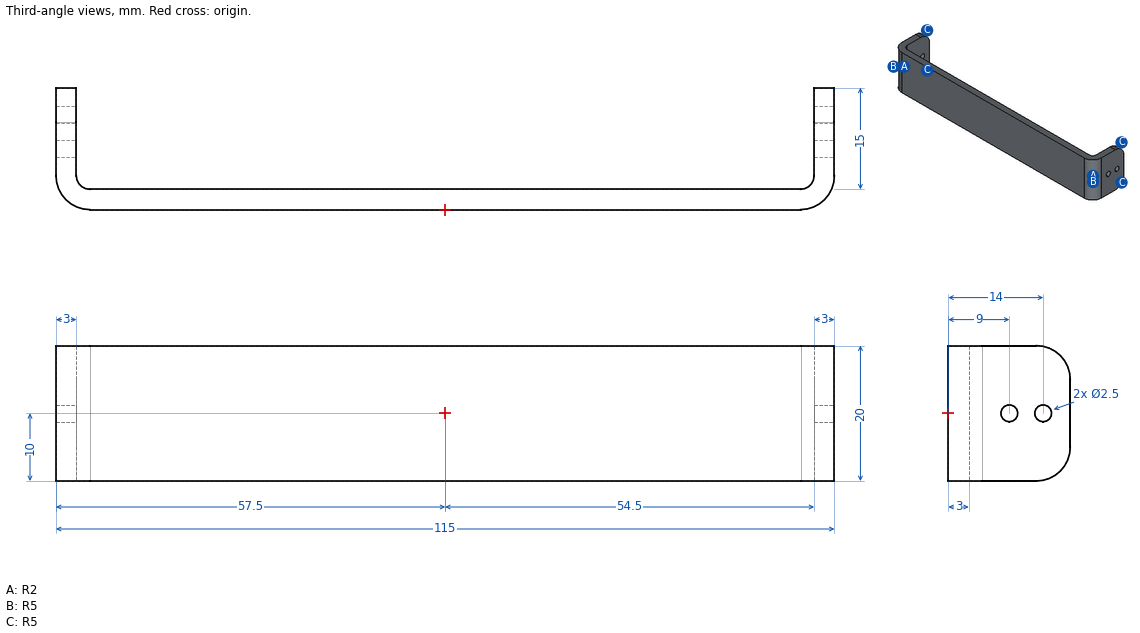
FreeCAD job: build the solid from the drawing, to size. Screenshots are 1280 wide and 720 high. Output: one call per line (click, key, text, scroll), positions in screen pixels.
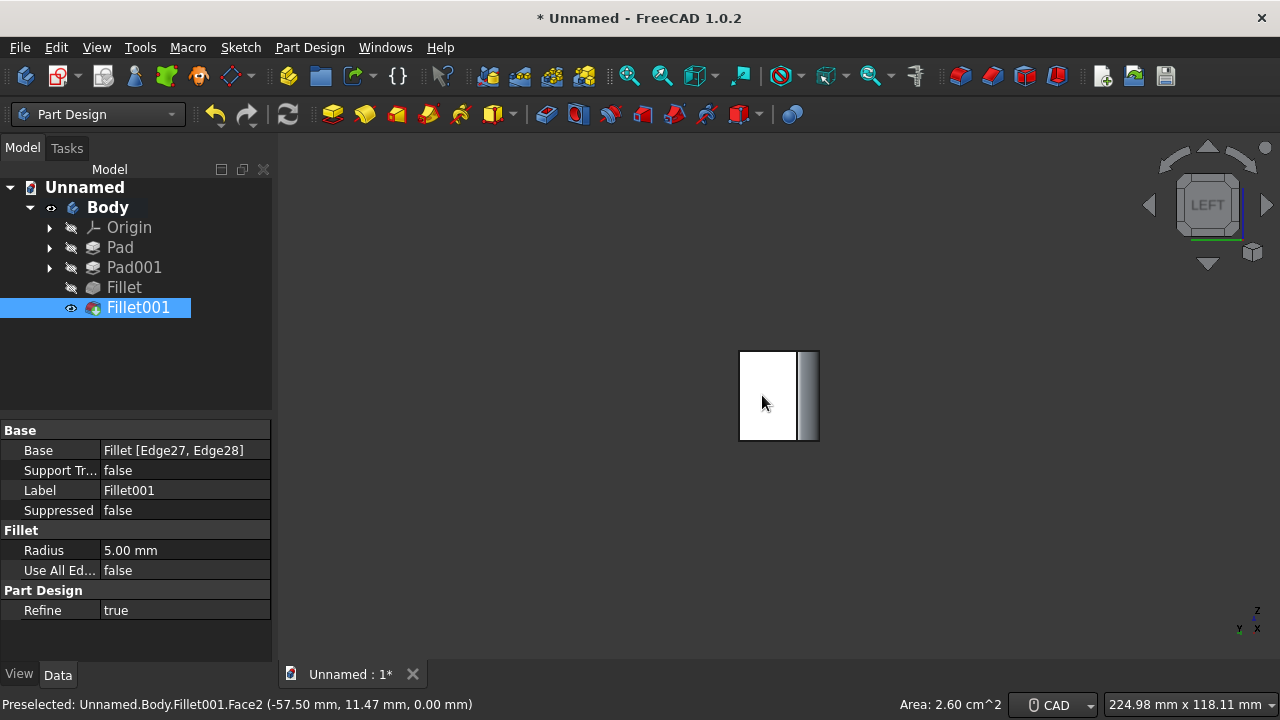
click(58, 76)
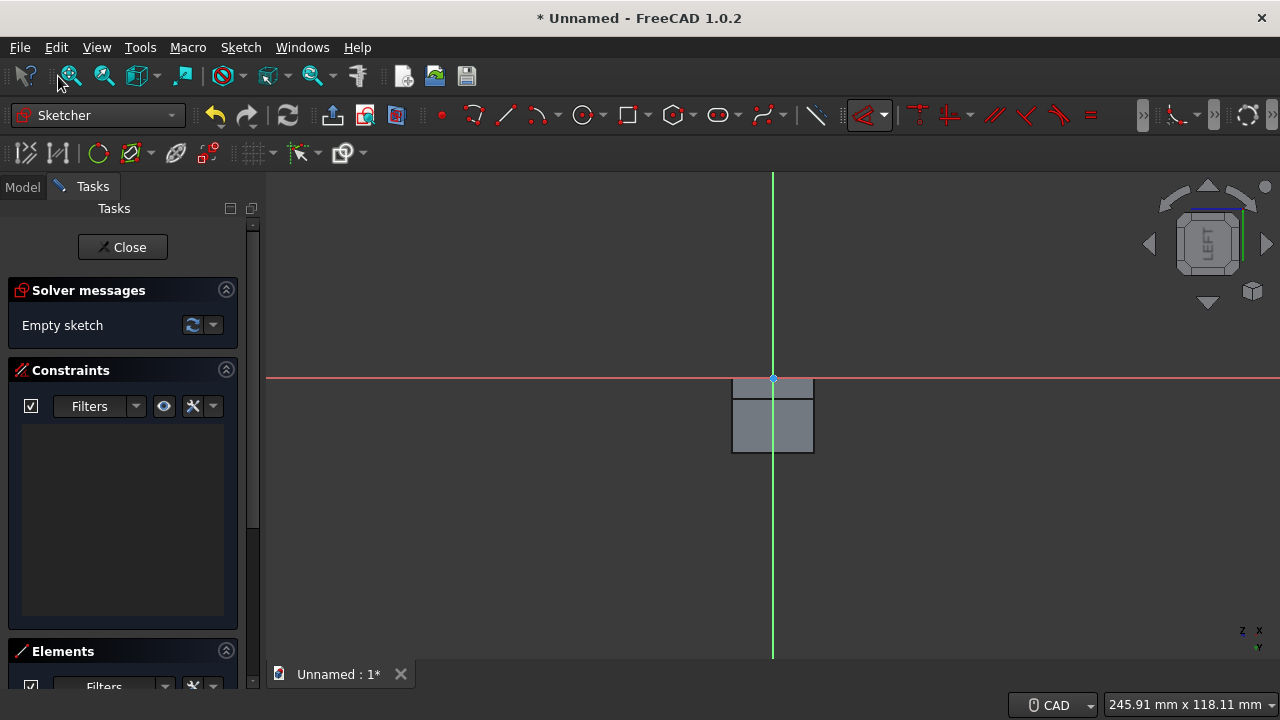
scroll(790, 408, up, 8)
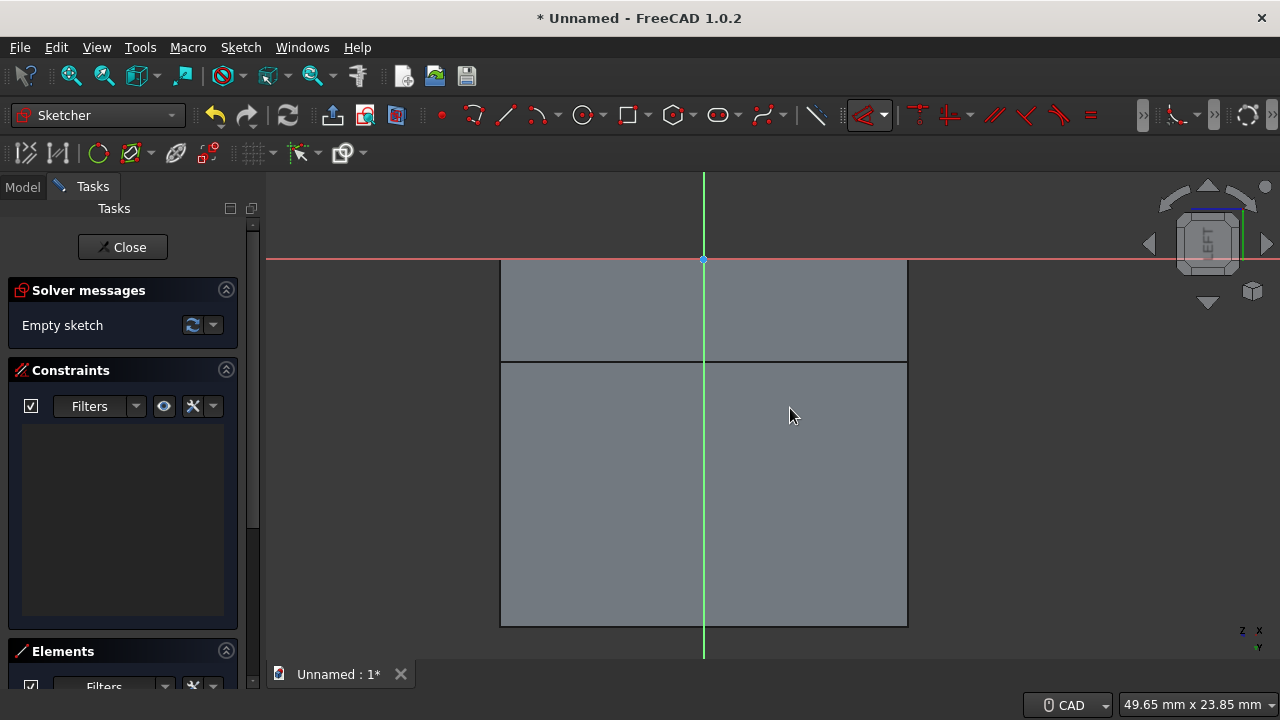
click(584, 116)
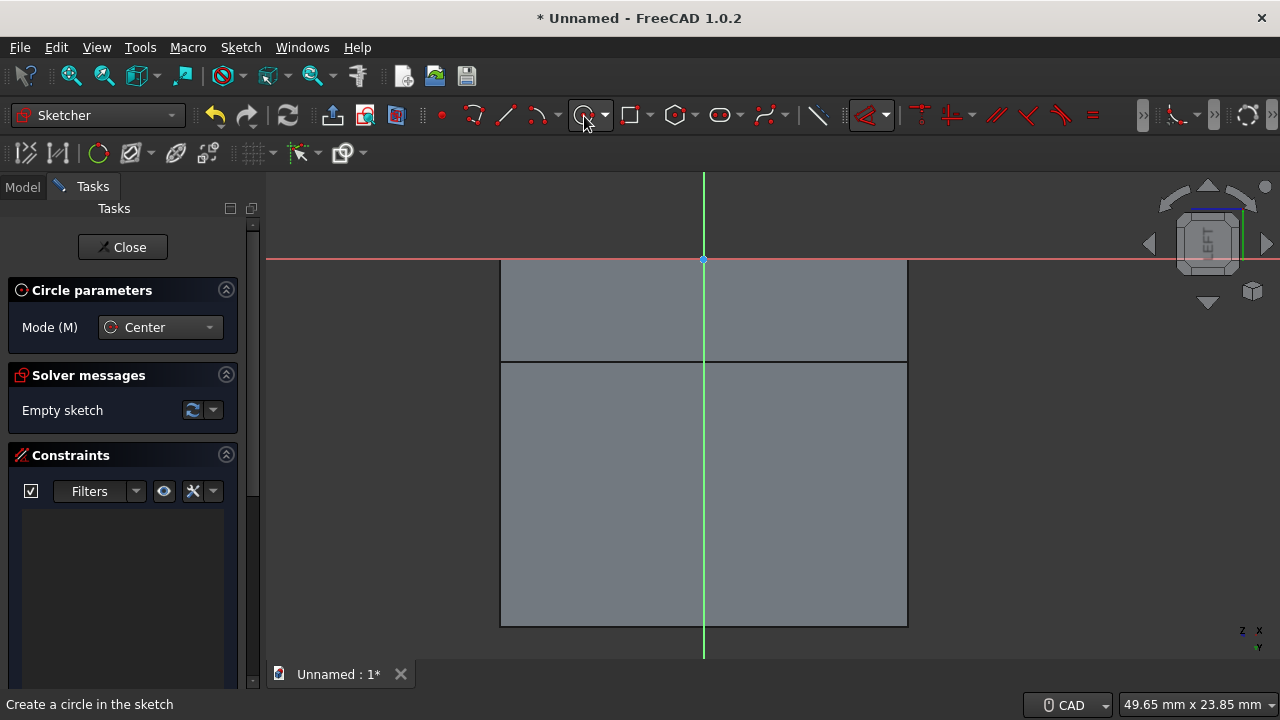
click(704, 545)
move(722, 527)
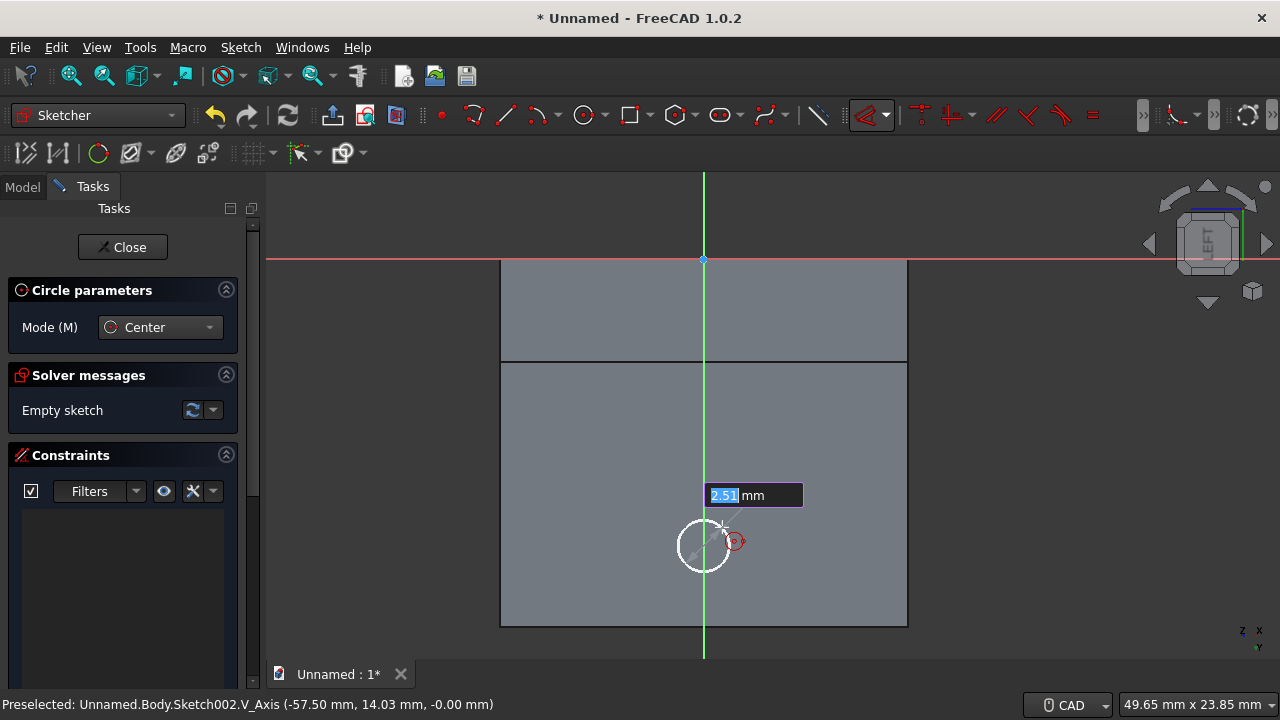
text(2.5)
key(Return)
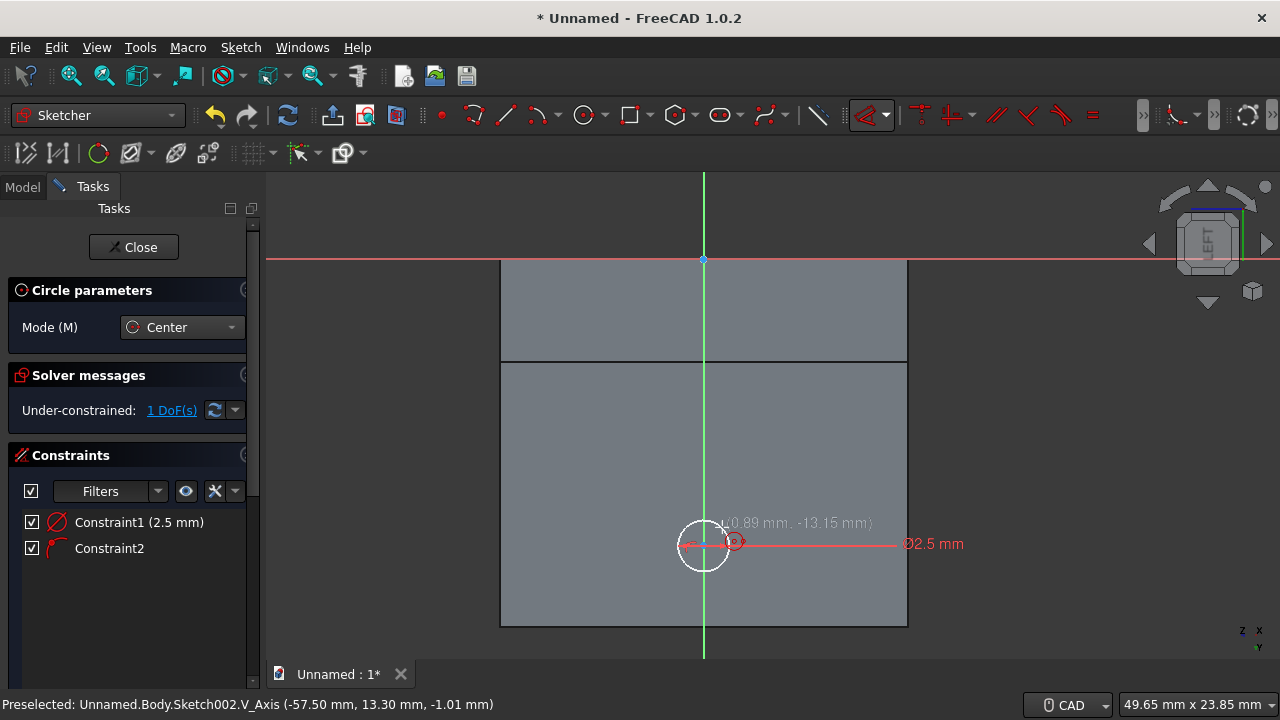
click(704, 443)
move(722, 425)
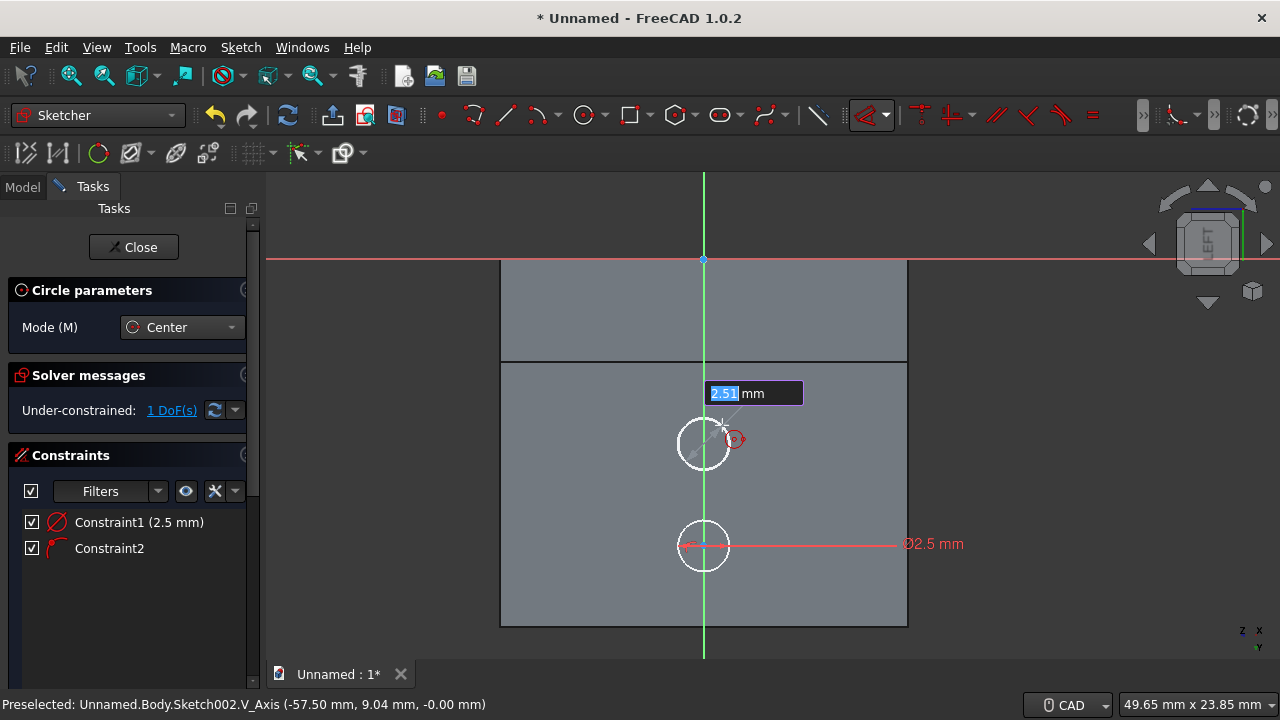
text(2.5)
key(Return)
key(Escape)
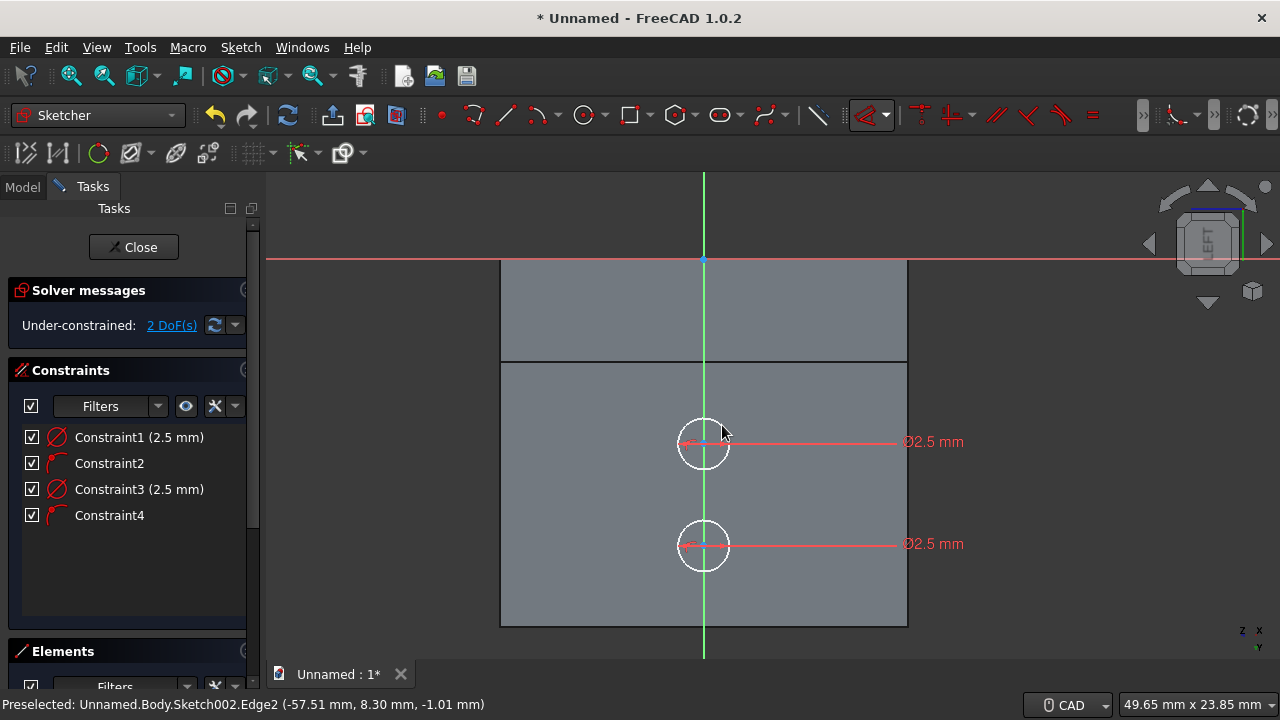
click(704, 444)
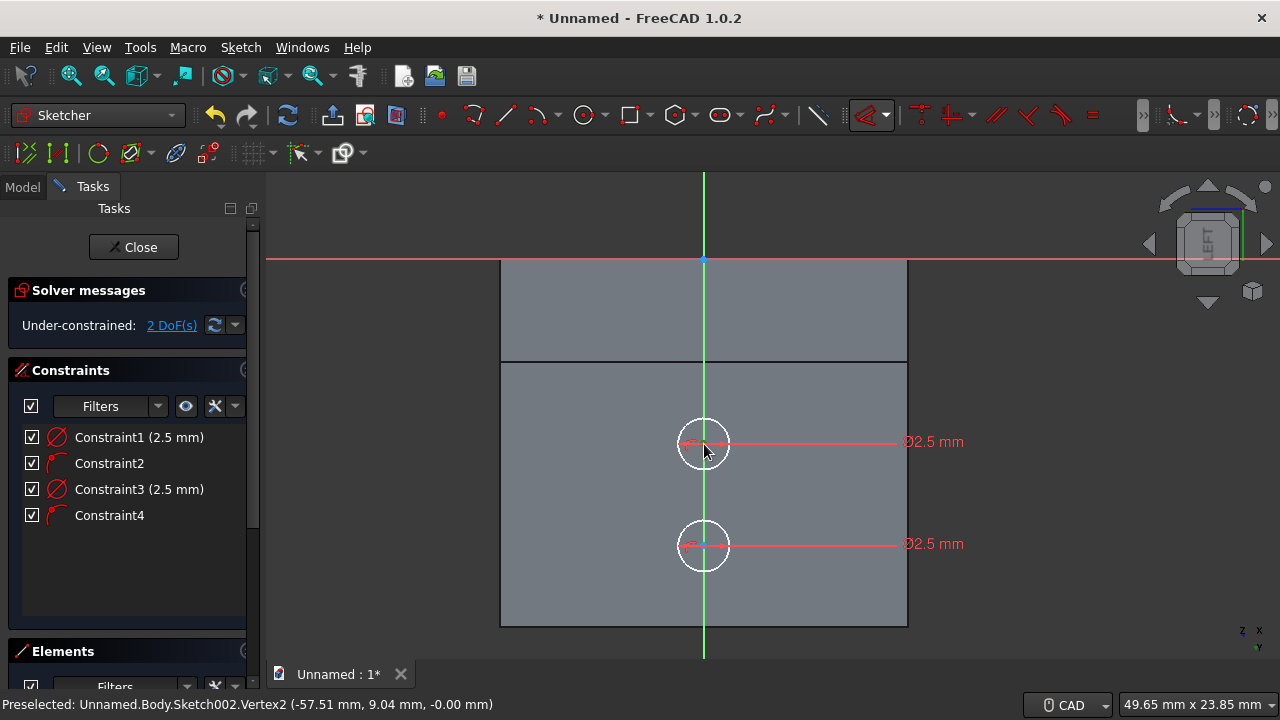
key(i)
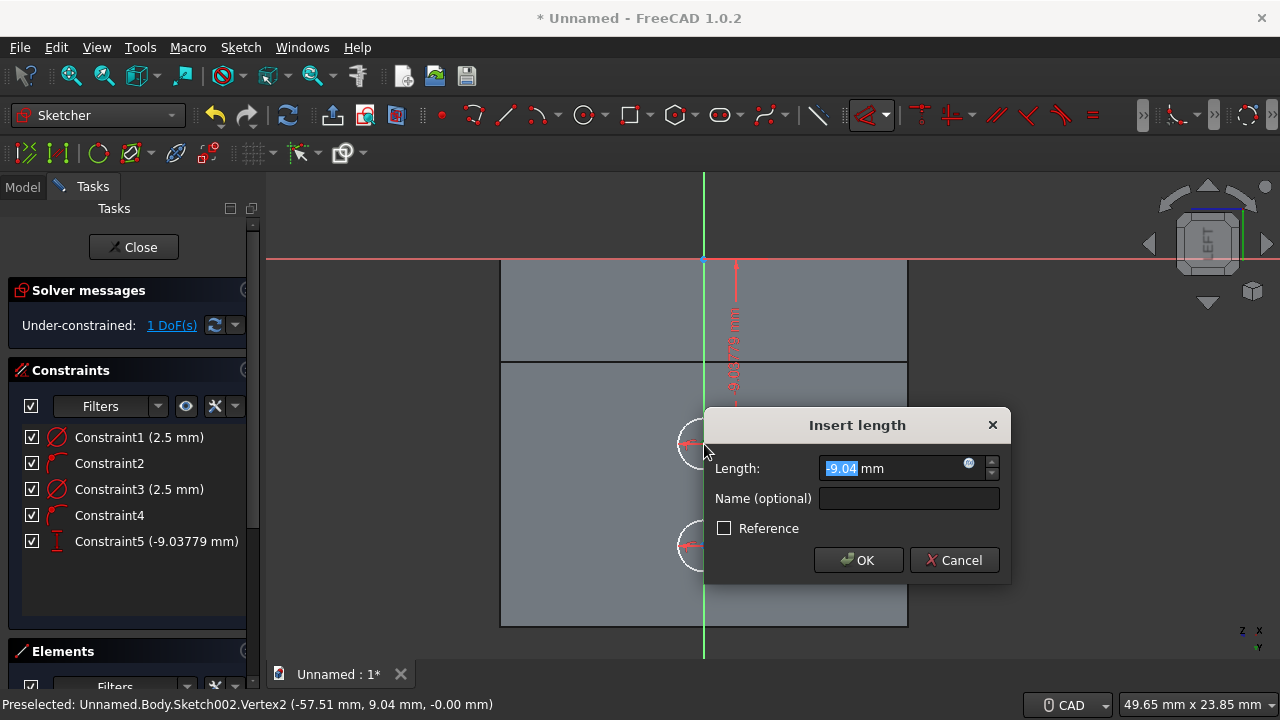
text(-9)
key(Return)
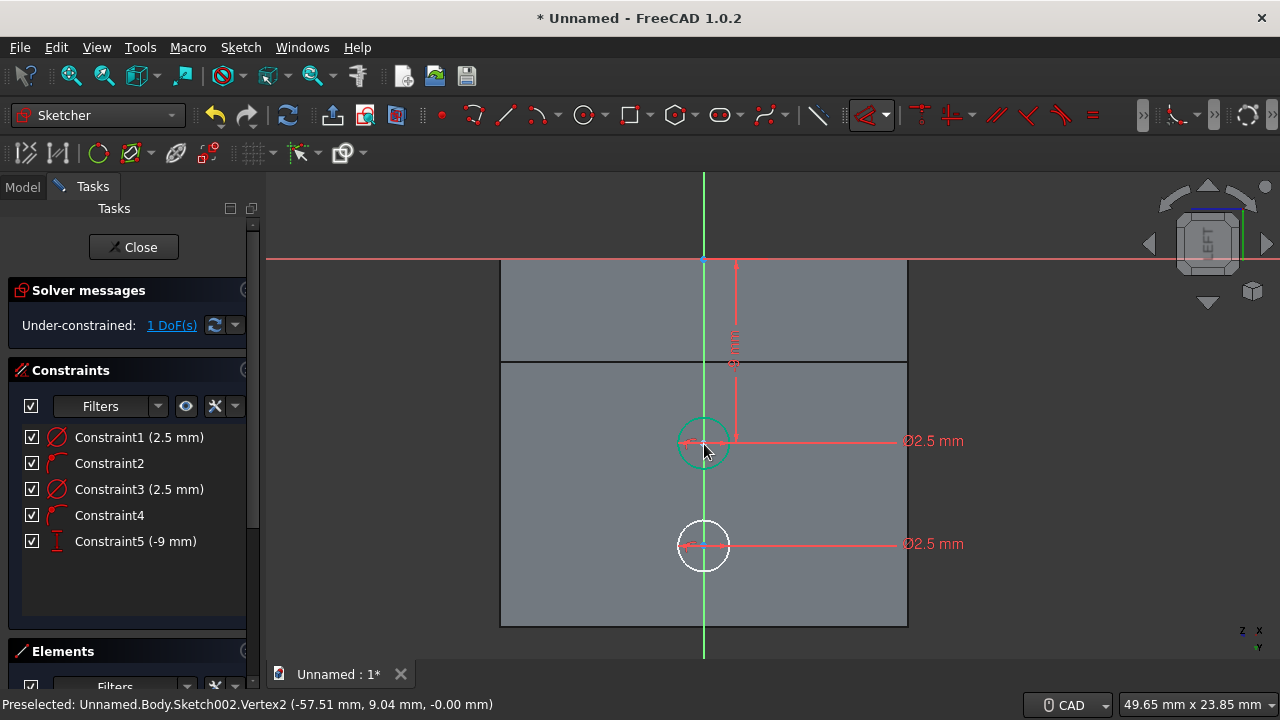
click(704, 546)